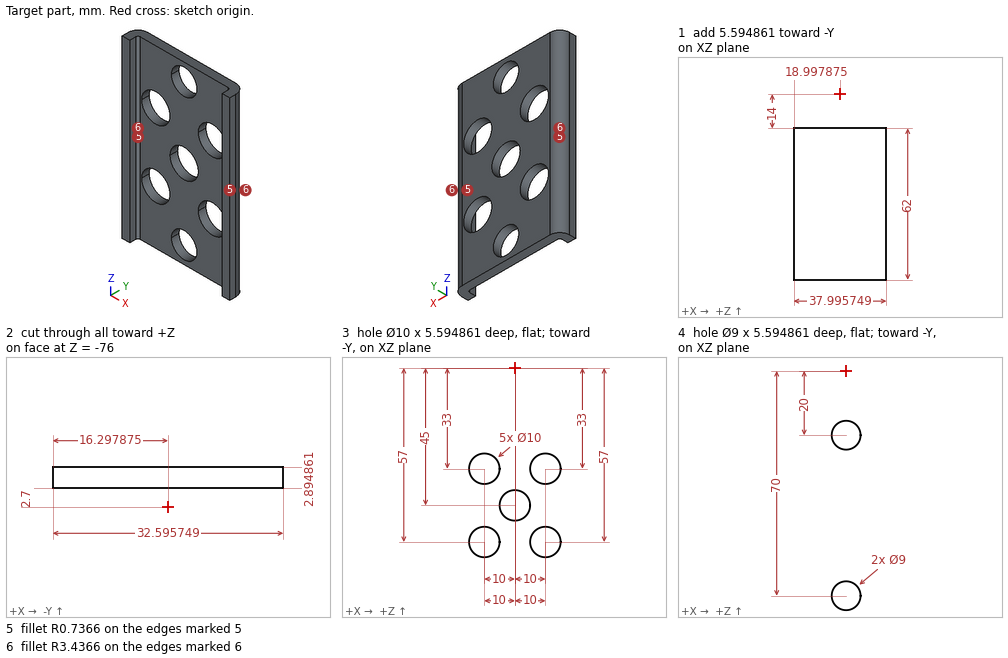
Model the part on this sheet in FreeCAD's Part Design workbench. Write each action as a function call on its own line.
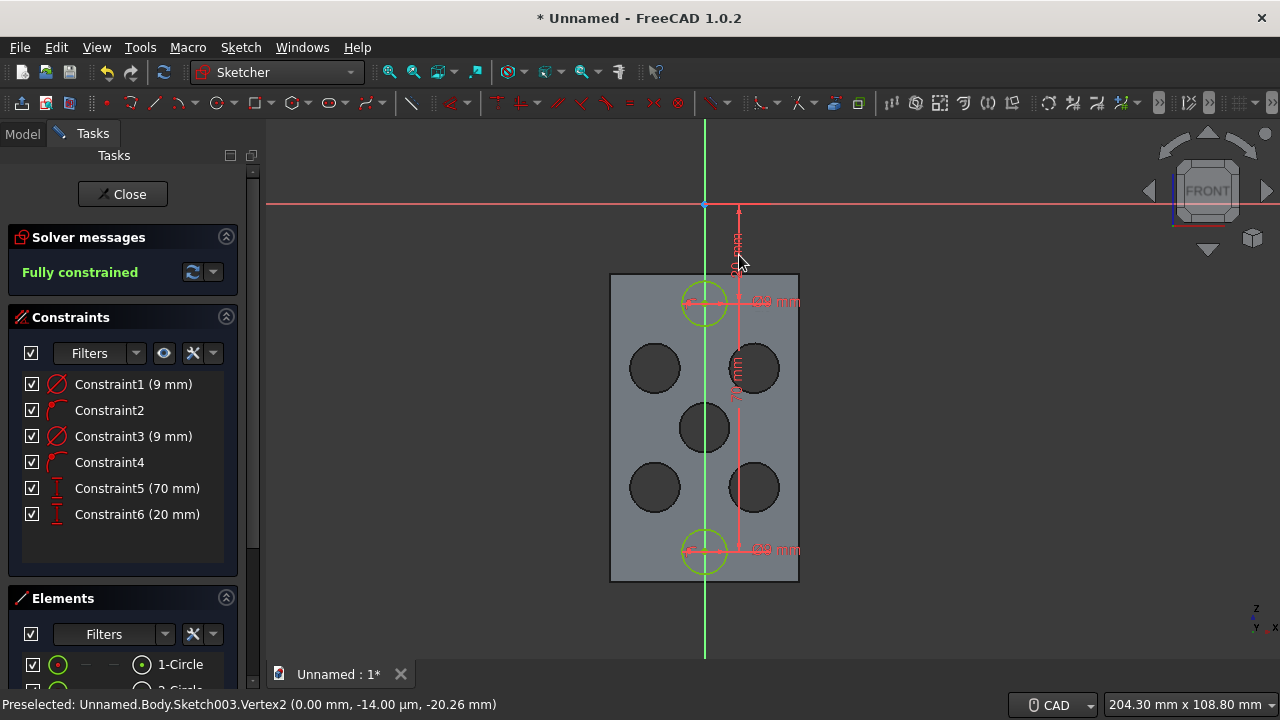
click(123, 194)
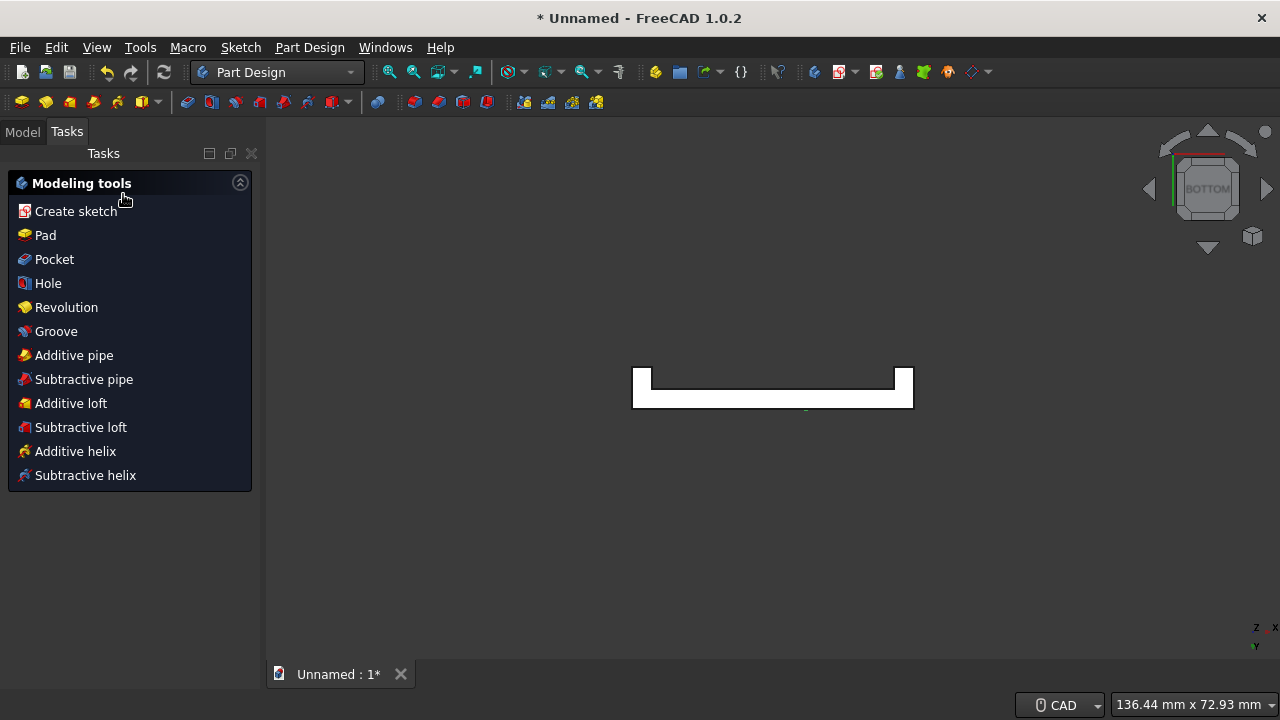
click(212, 102)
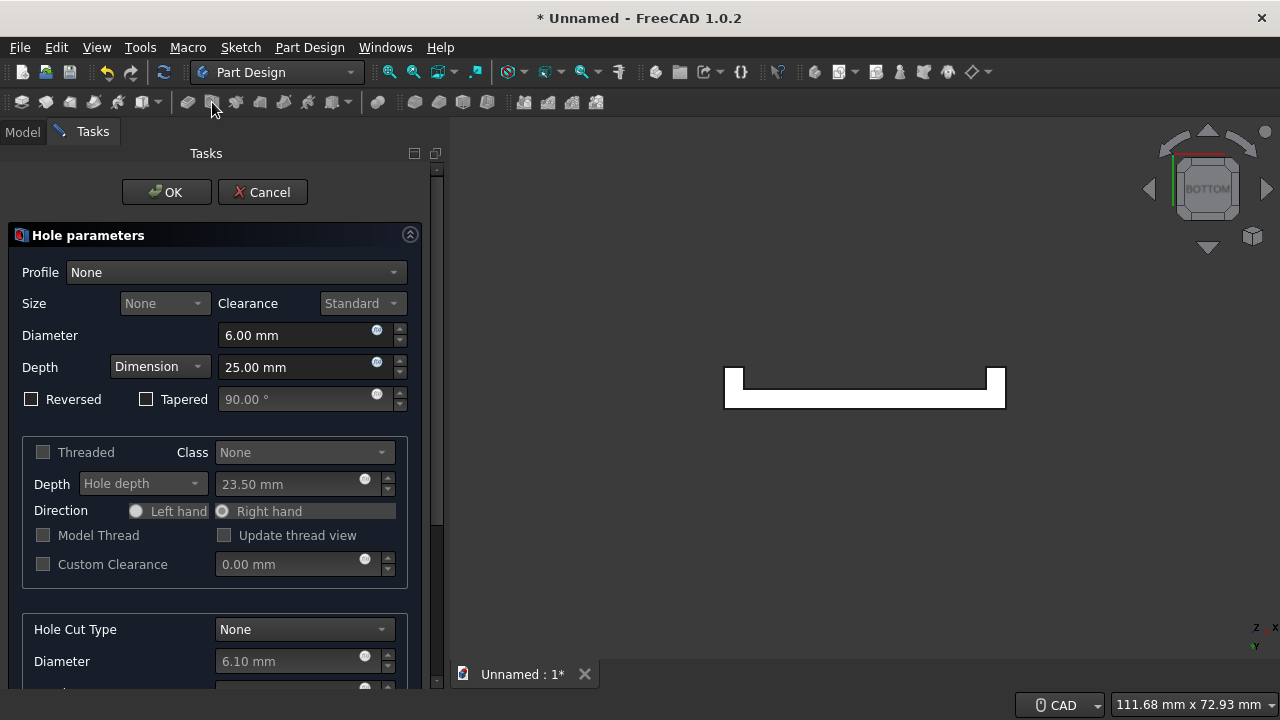
triple_click(305, 335)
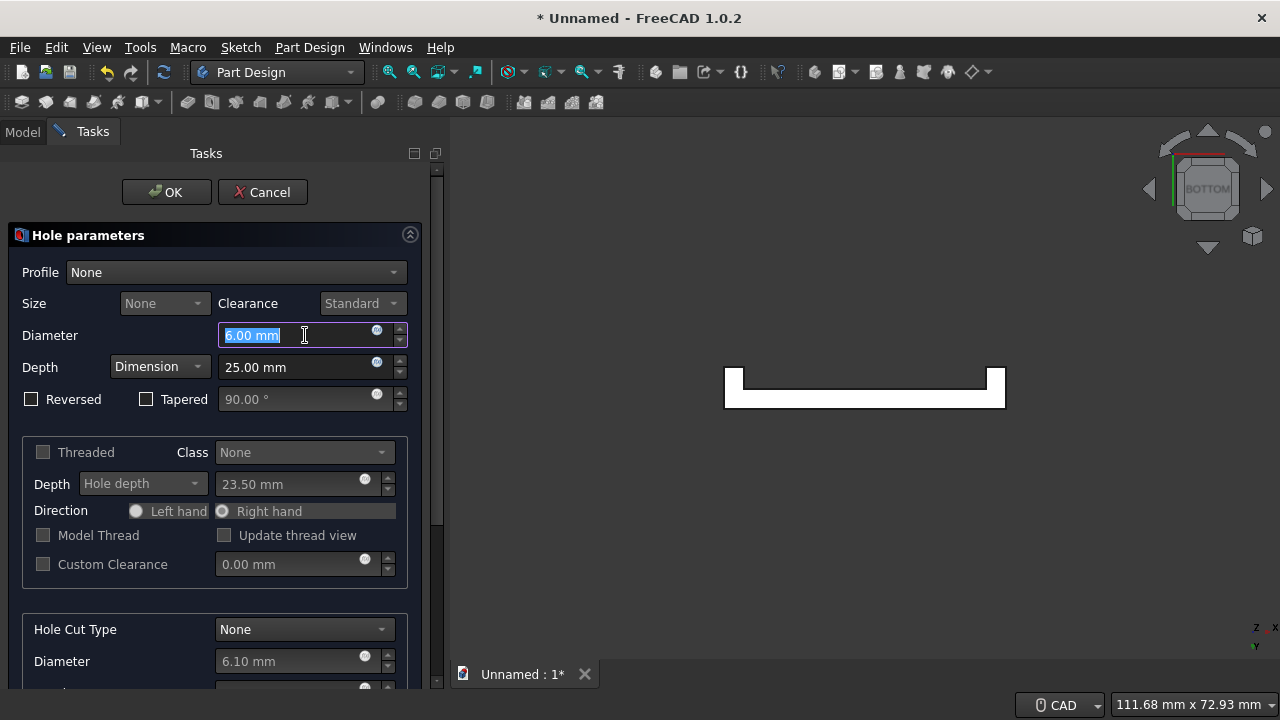
text(9)
key(Tab)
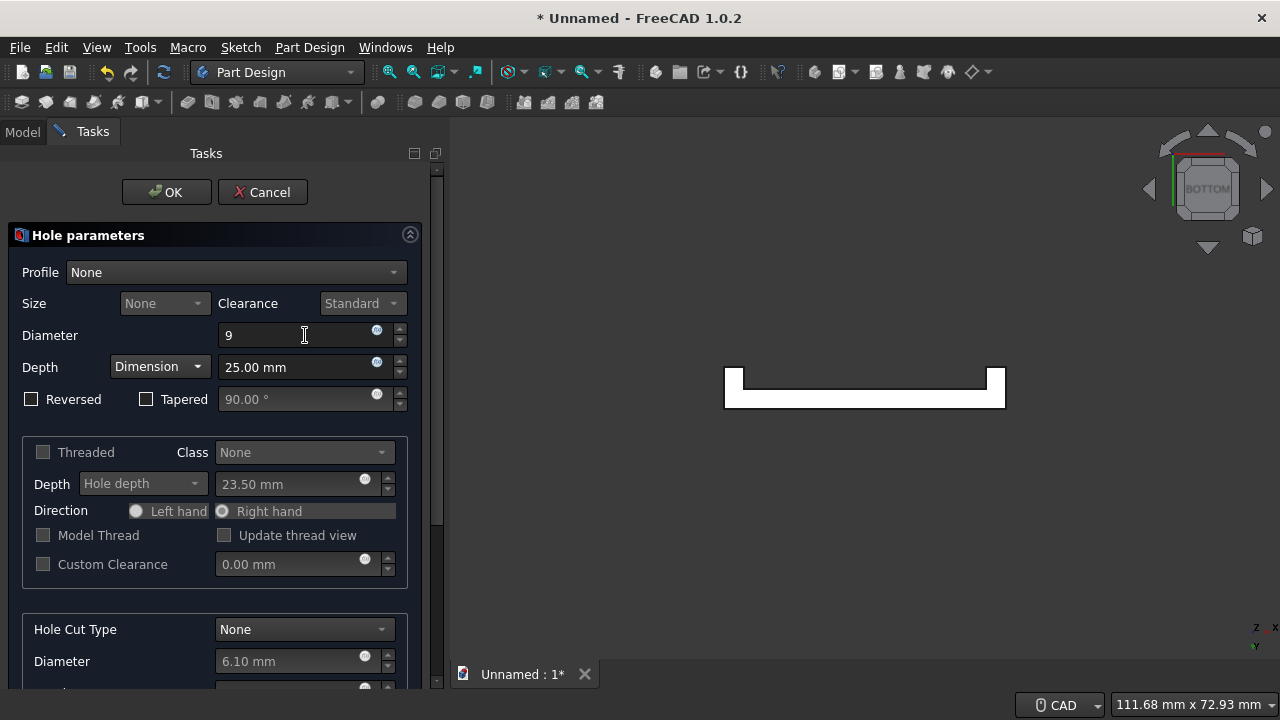
triple_click(305, 367)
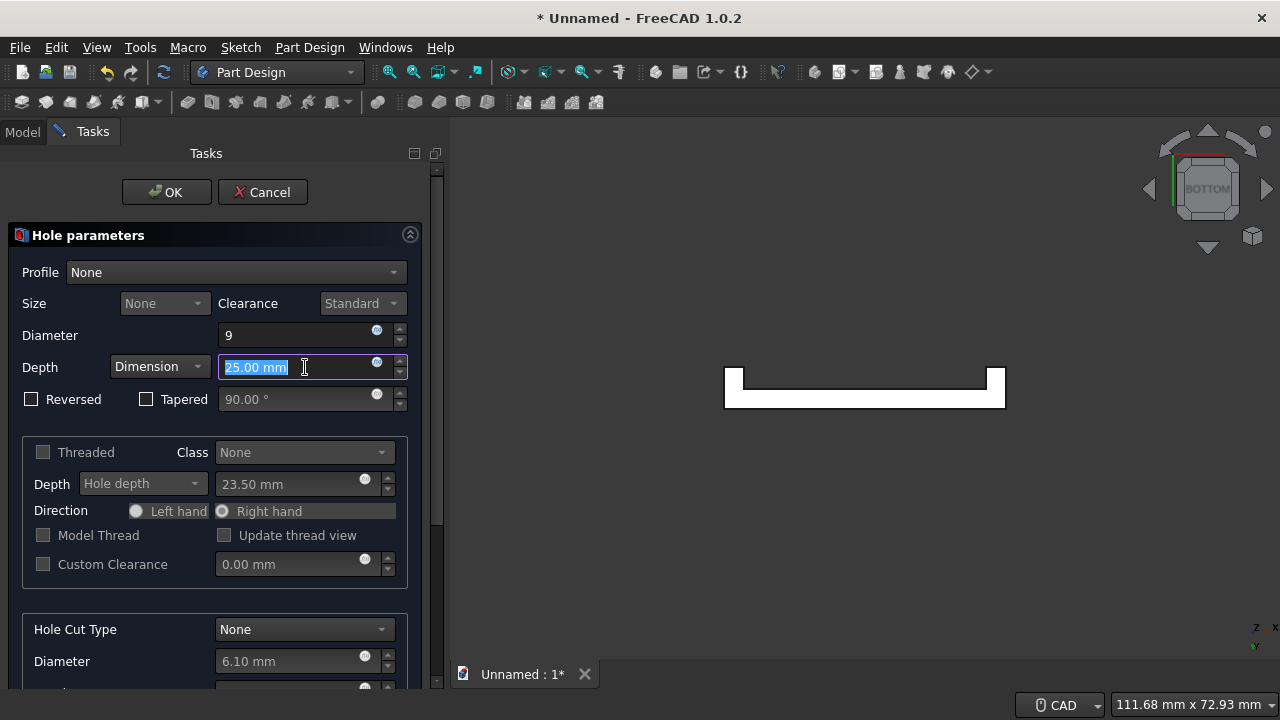
text(5.594861)
key(Tab)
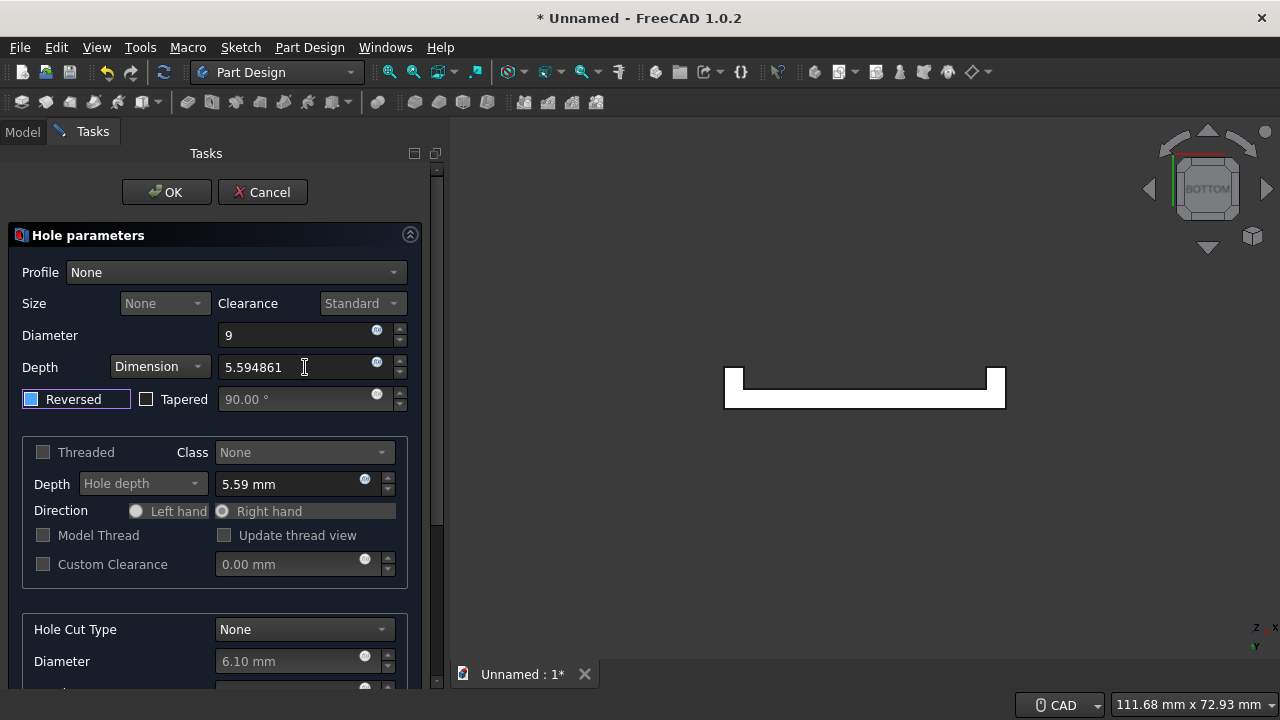
click(30, 399)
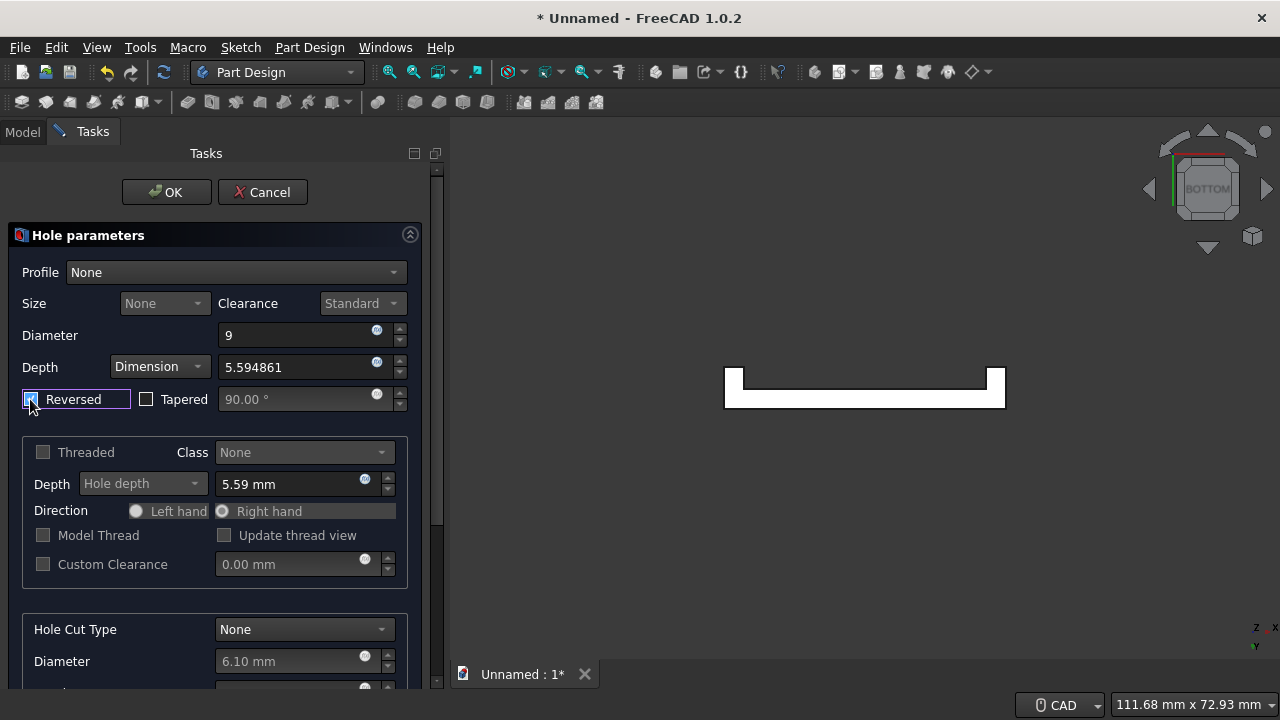
scroll(437, 426, down, 4)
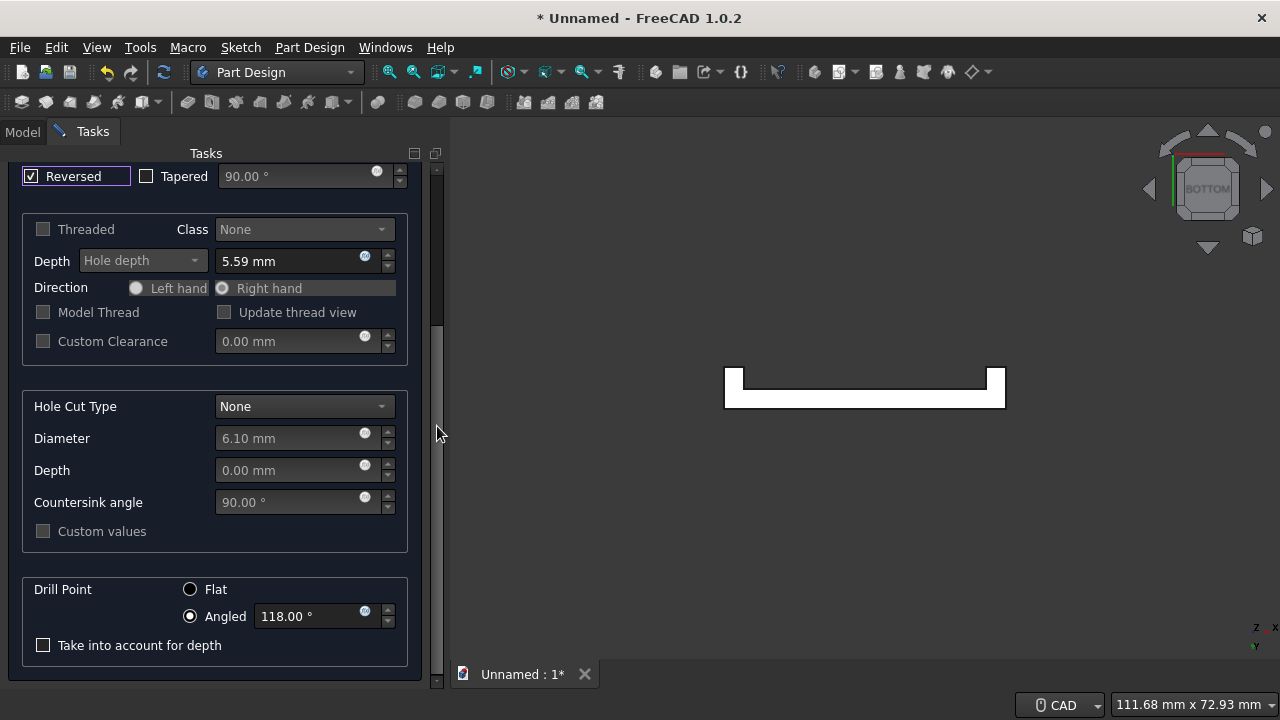
click(191, 589)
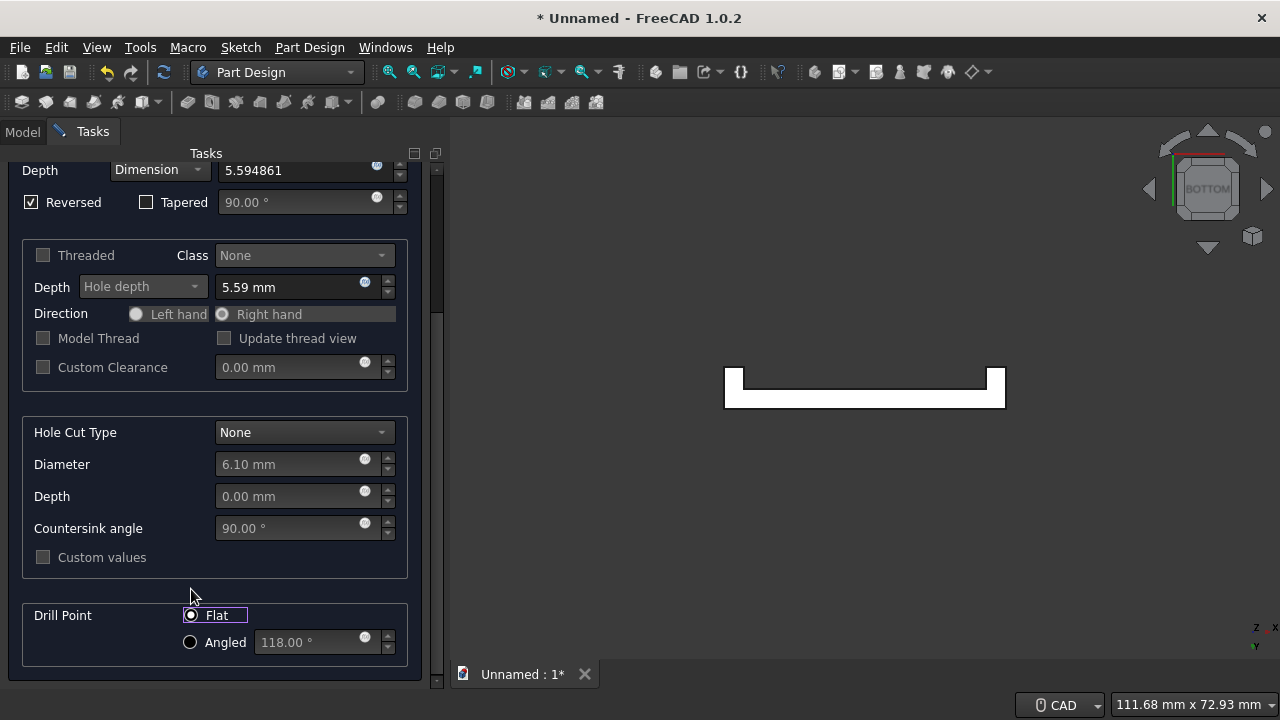
scroll(437, 426, up, 5)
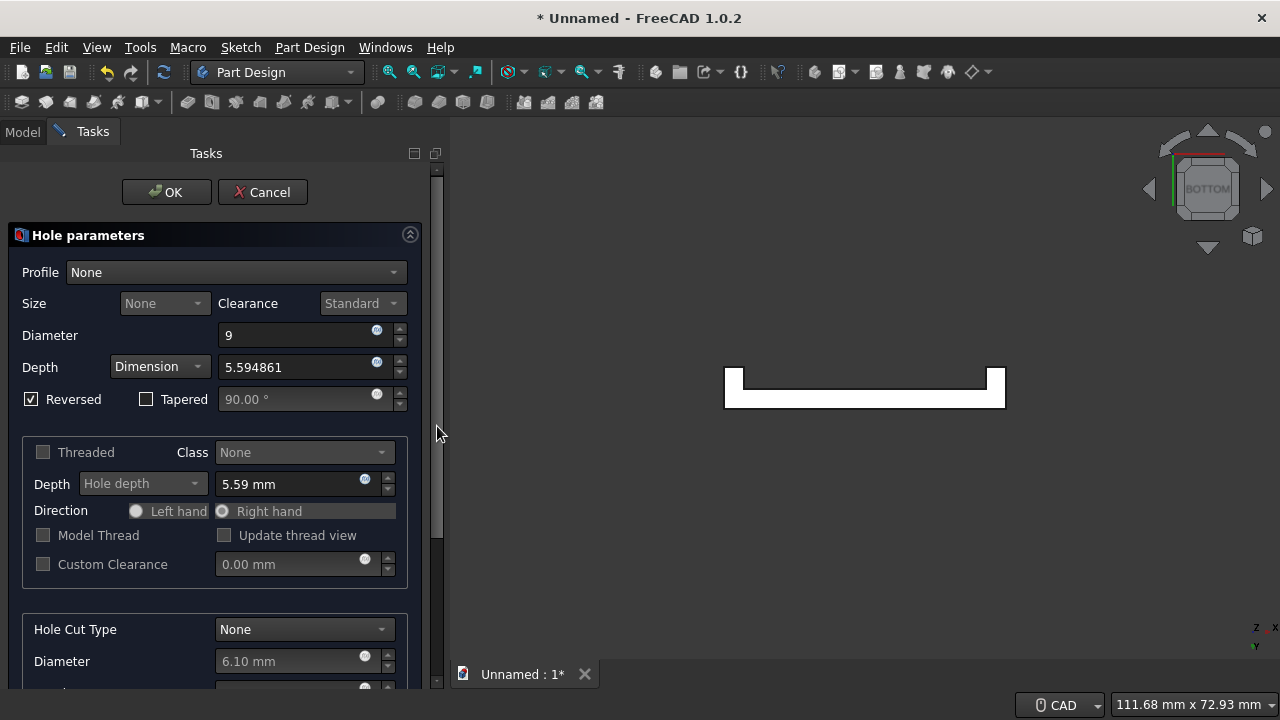
click(167, 192)